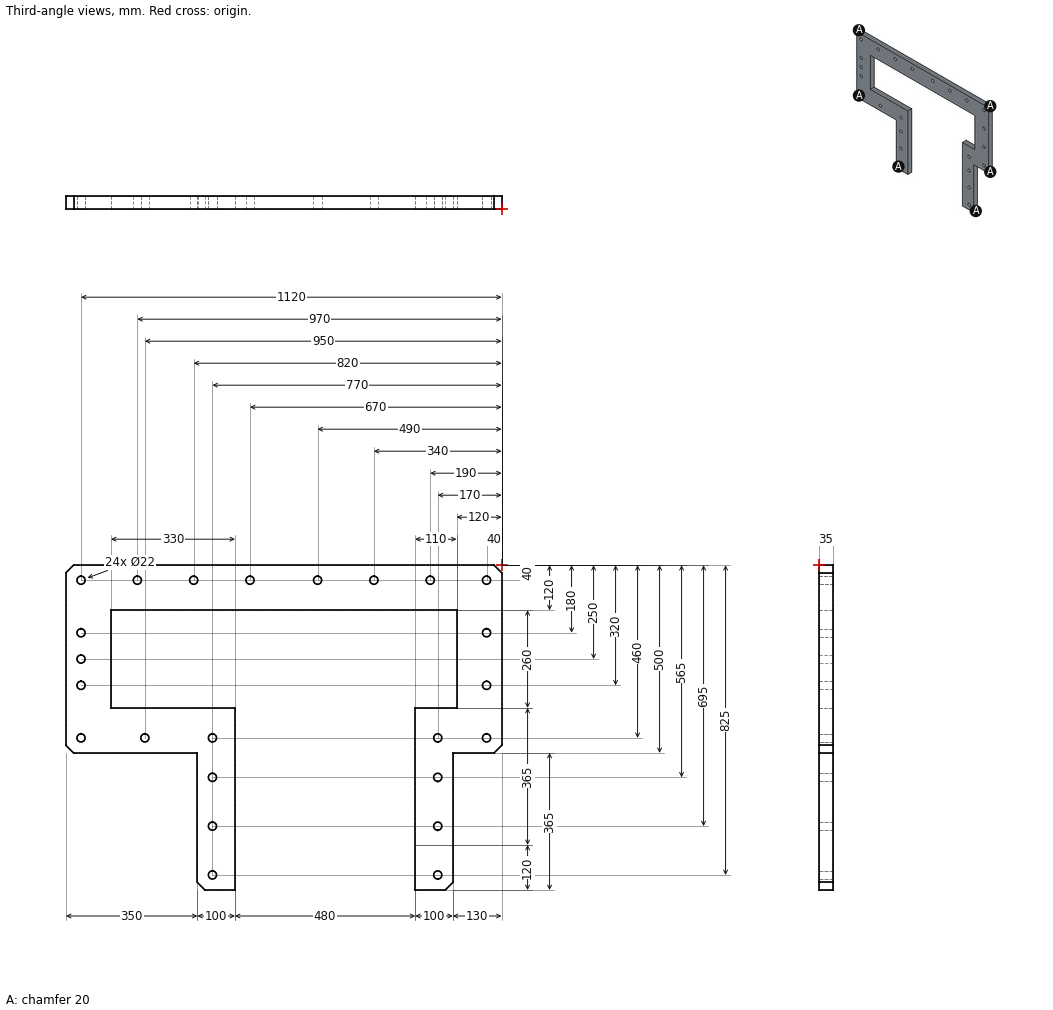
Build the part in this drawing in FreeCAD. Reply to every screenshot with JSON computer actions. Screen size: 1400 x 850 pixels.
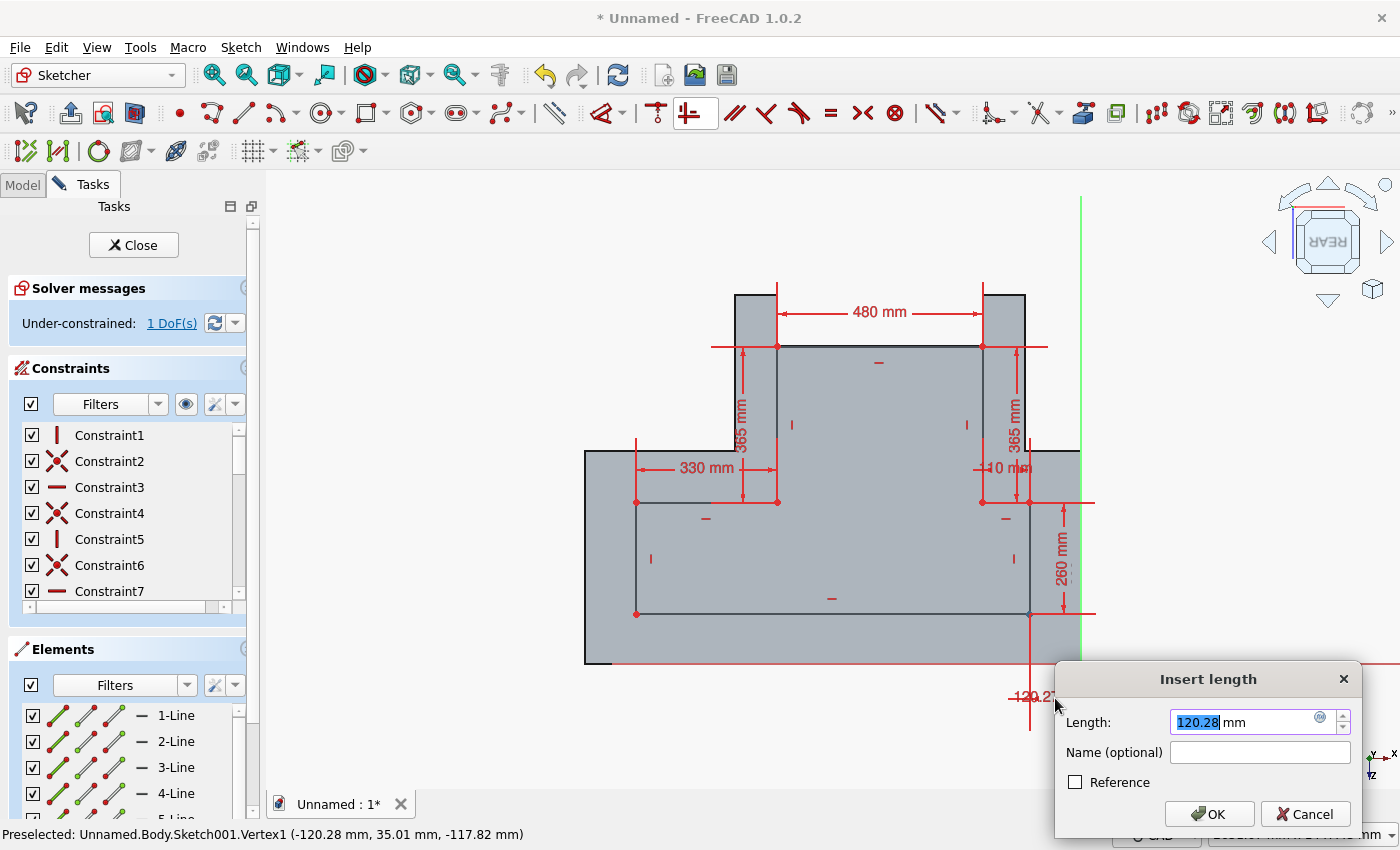
{"action": "type", "text": "120"}
{"action": "key", "text": "Return"}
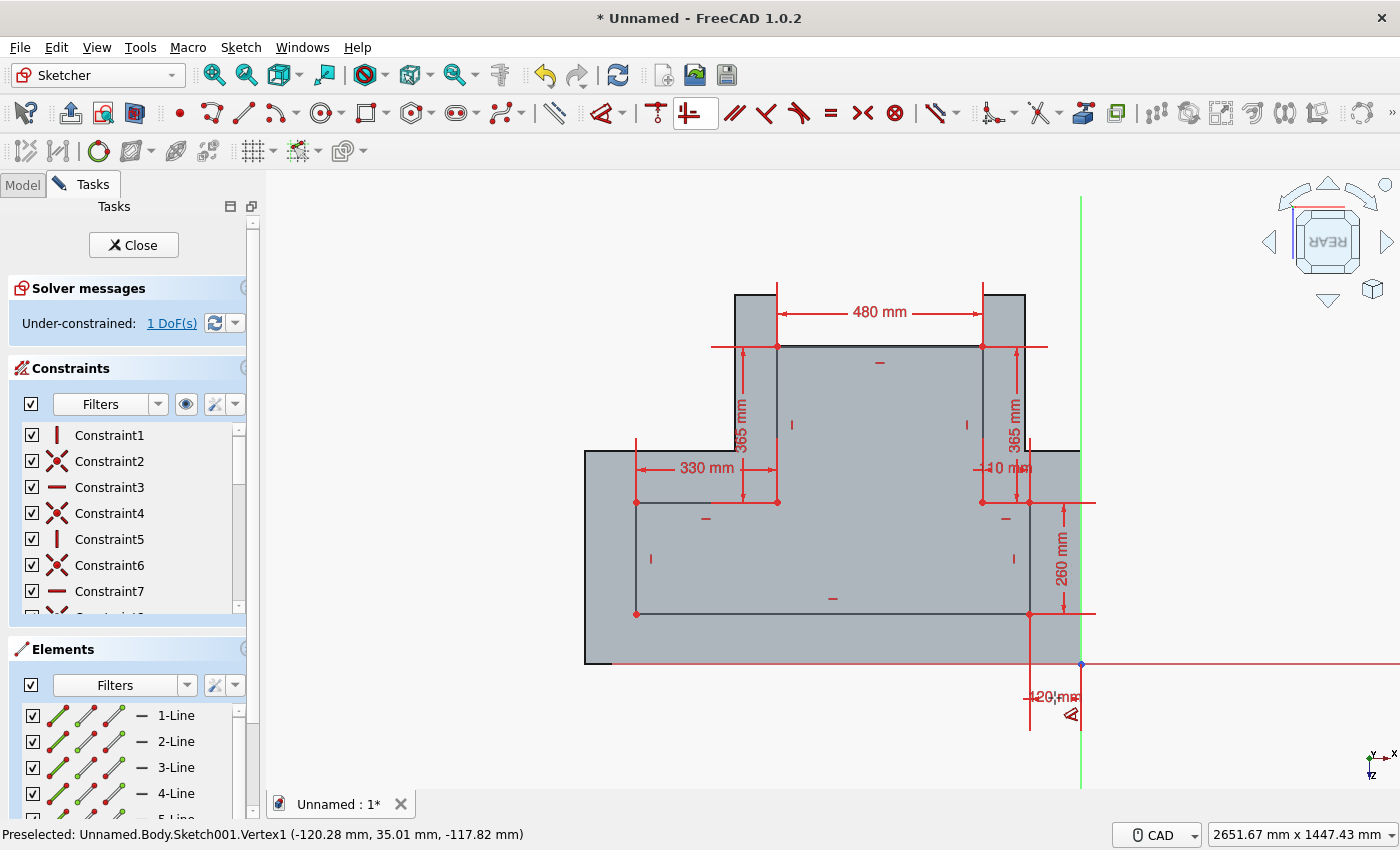
{"action": "left_click", "coordinate": [1030, 614]}
{"action": "left_click", "coordinate": [1115, 639]}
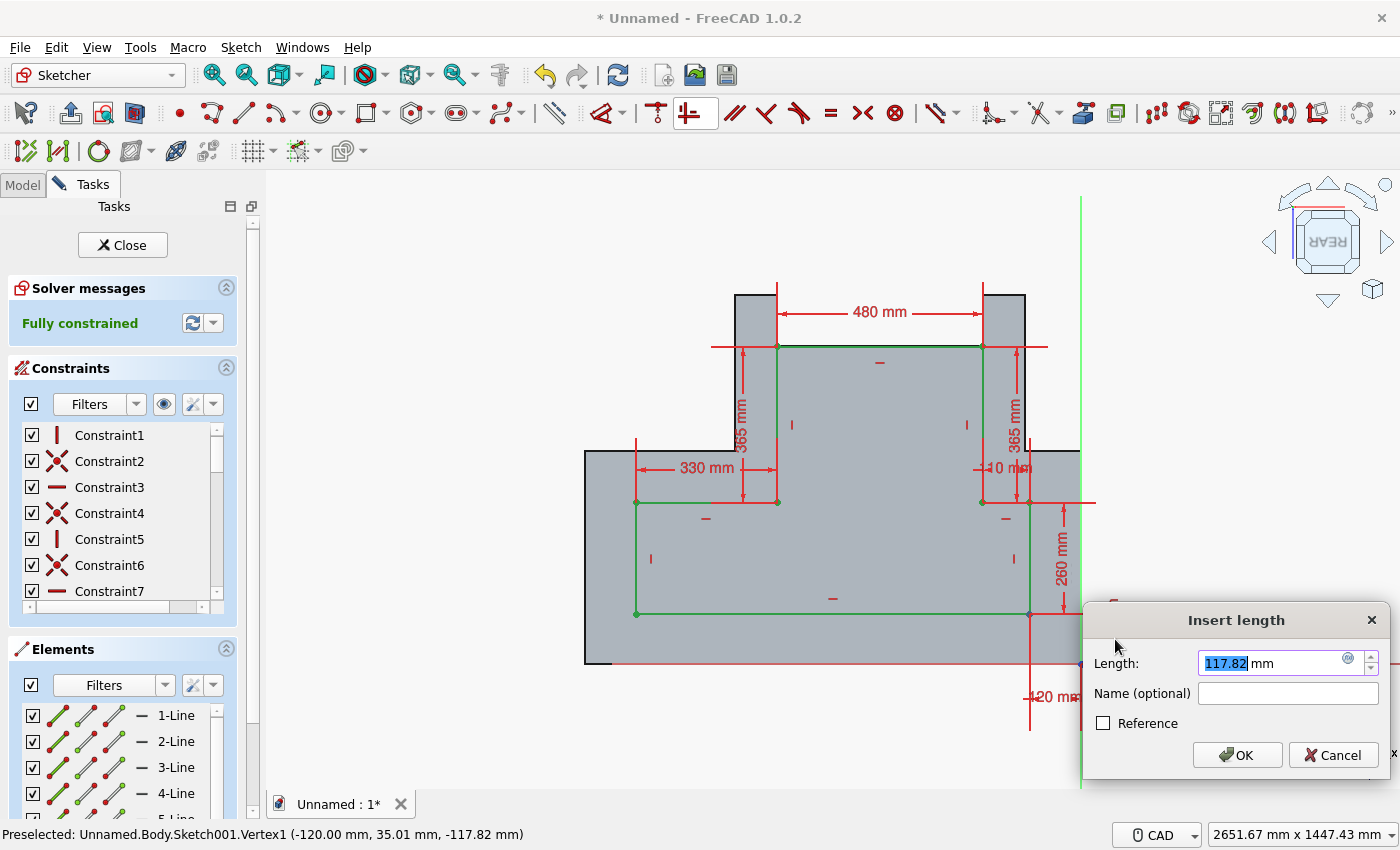
{"action": "type", "text": "120"}
{"action": "key", "text": "Return"}
{"action": "key", "text": "Escape"}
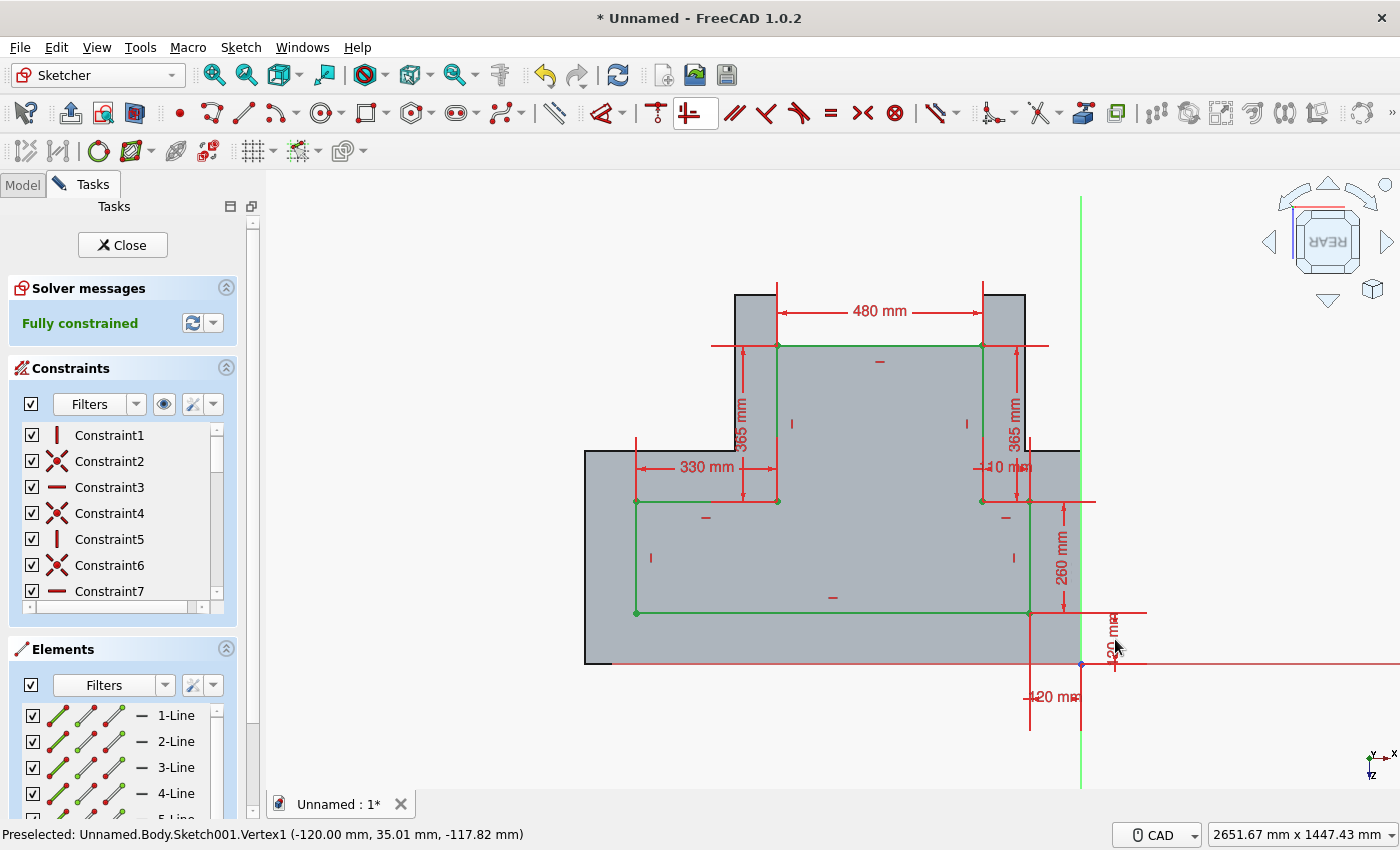
{"action": "left_click", "coordinate": [123, 245]}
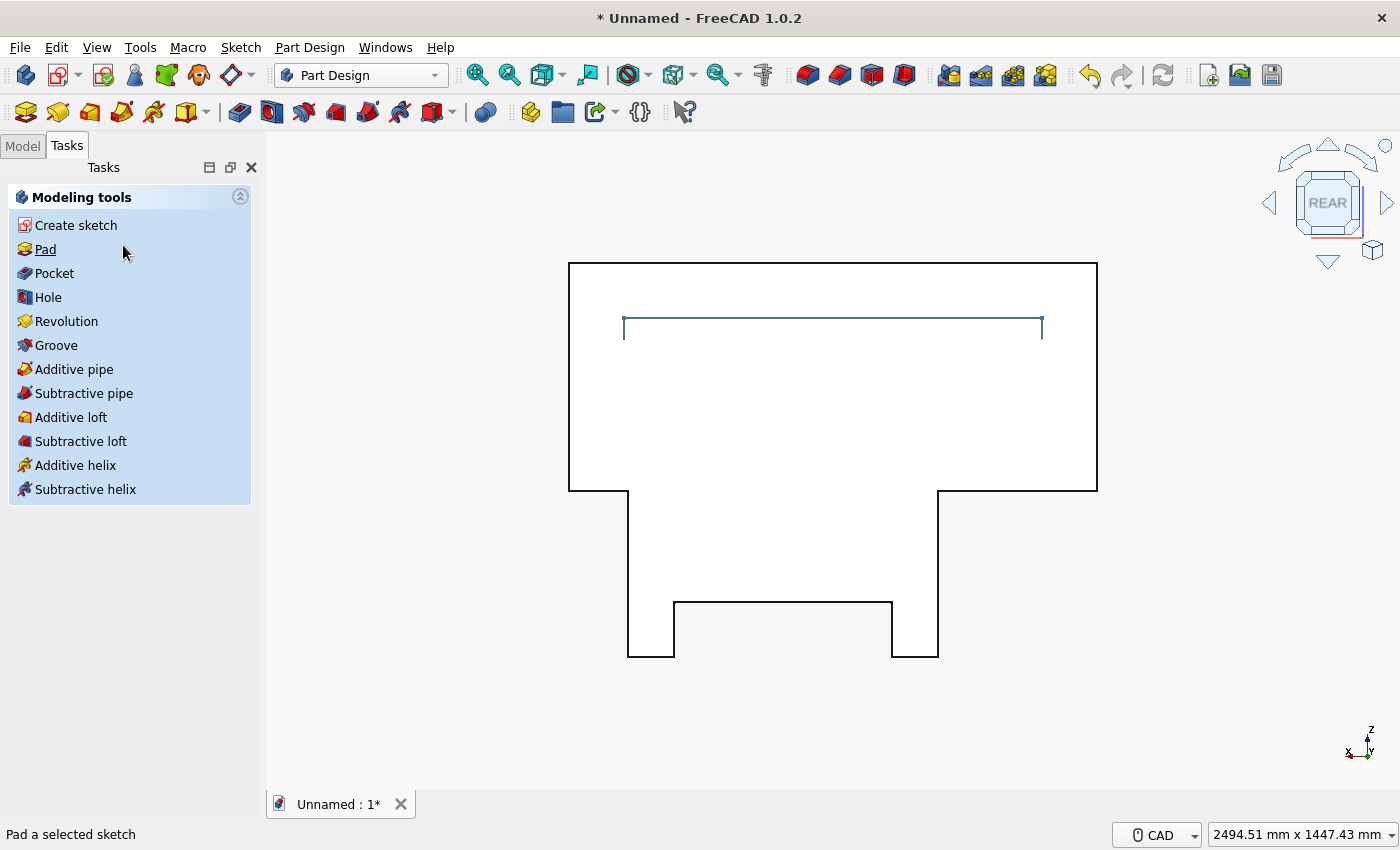
{"action": "left_click", "coordinate": [240, 112]}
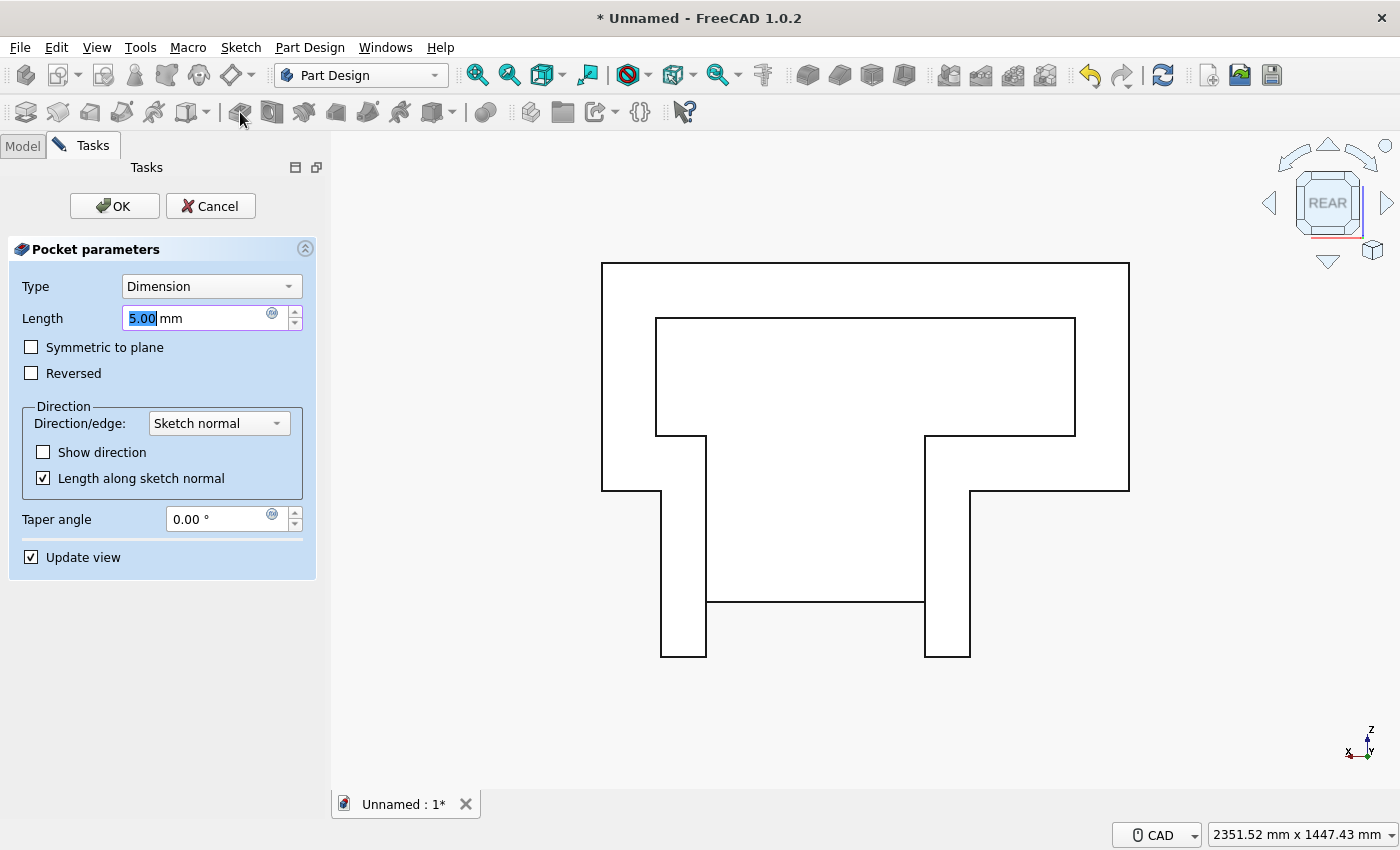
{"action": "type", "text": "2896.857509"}
{"action": "key", "text": "Tab"}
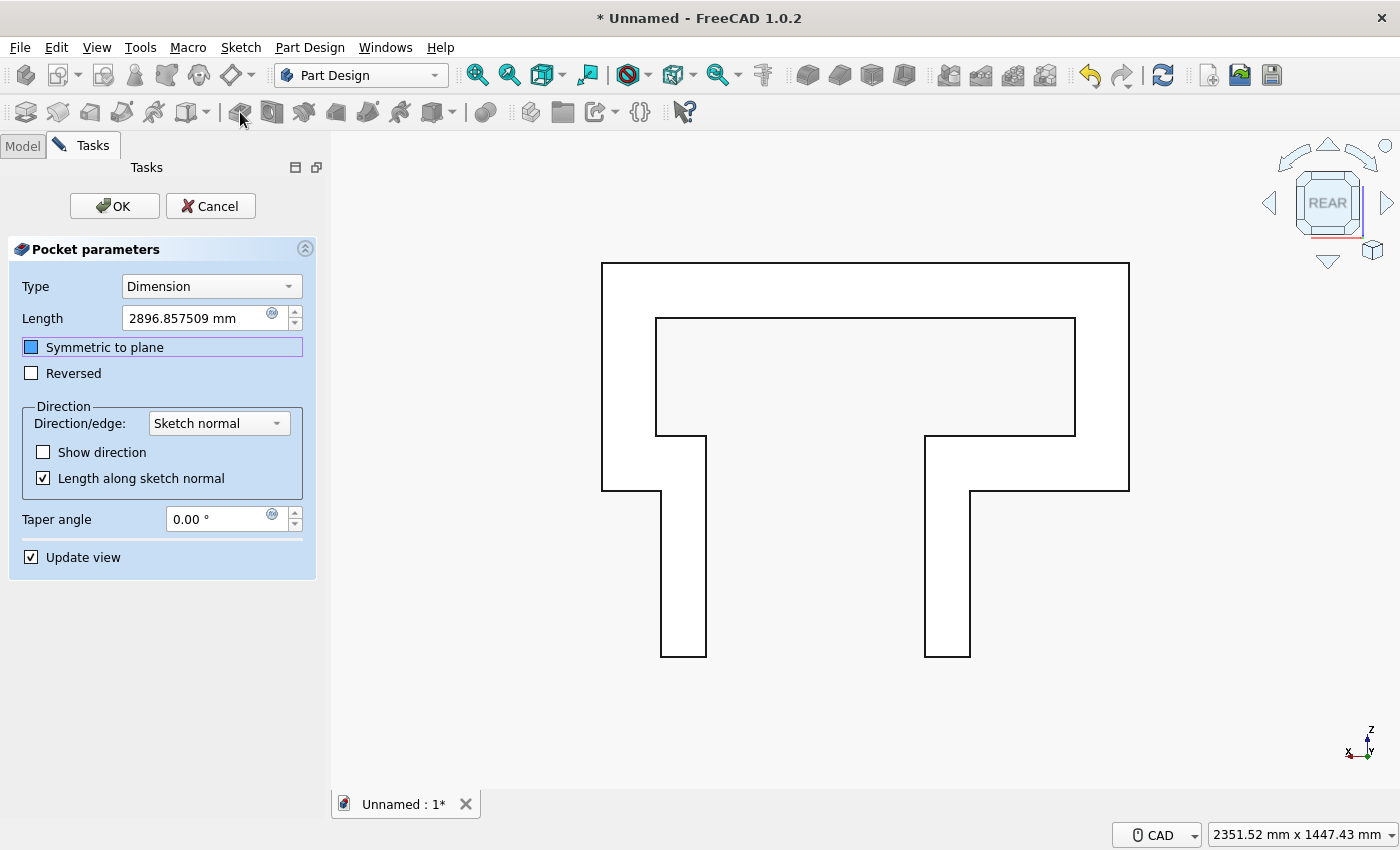
{"action": "left_click", "coordinate": [30, 347]}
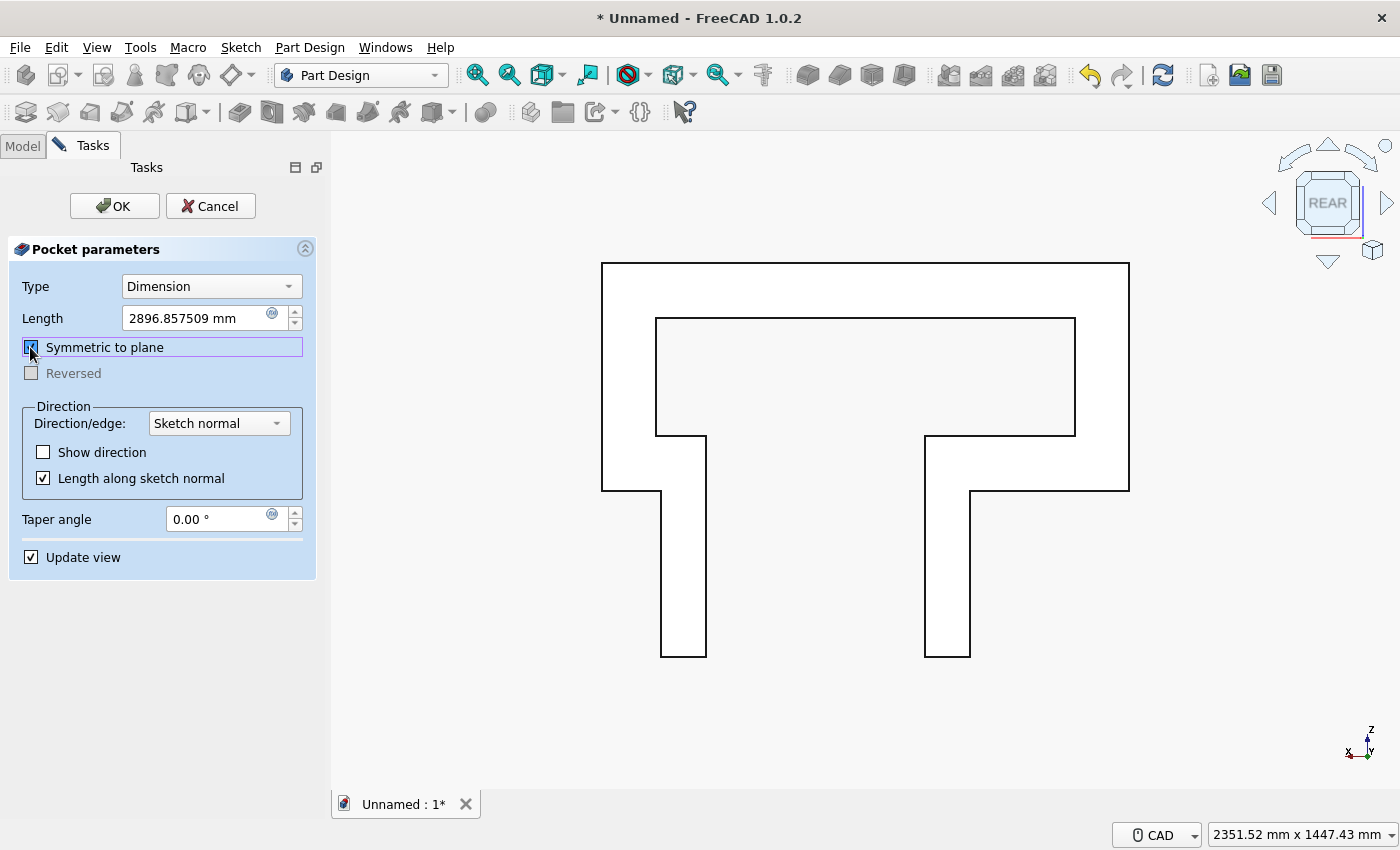
{"action": "left_click", "coordinate": [115, 206]}